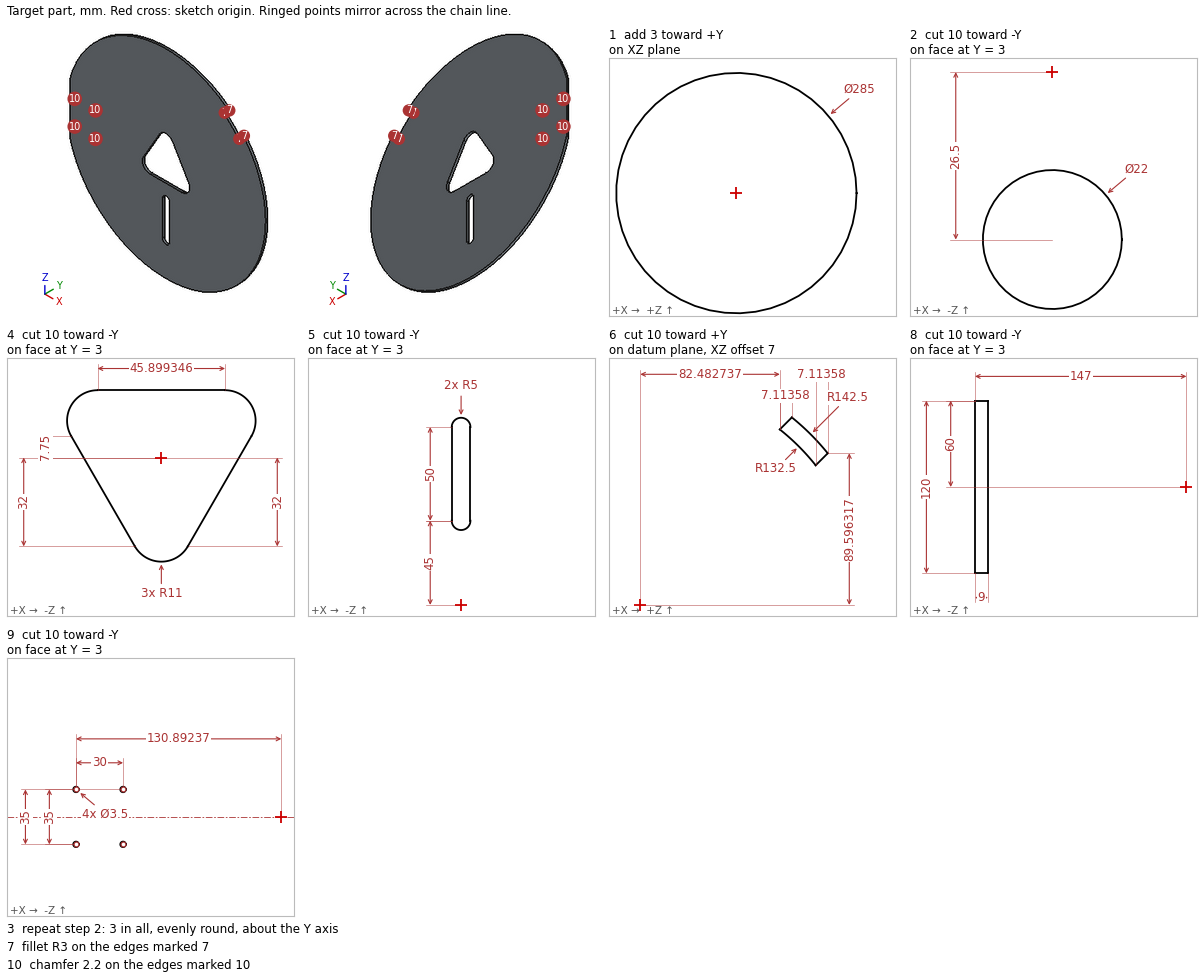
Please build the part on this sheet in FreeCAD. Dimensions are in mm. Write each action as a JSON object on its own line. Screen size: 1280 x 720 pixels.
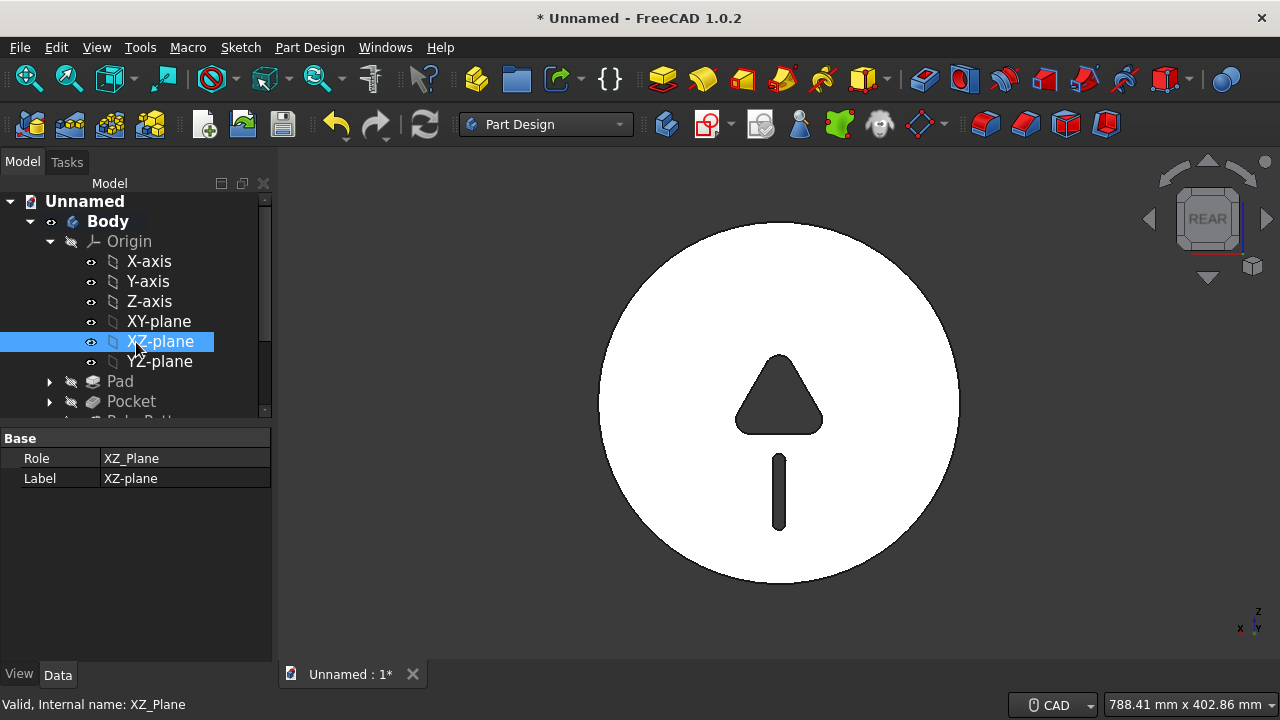
{"action": "left_click", "coordinate": [920, 124]}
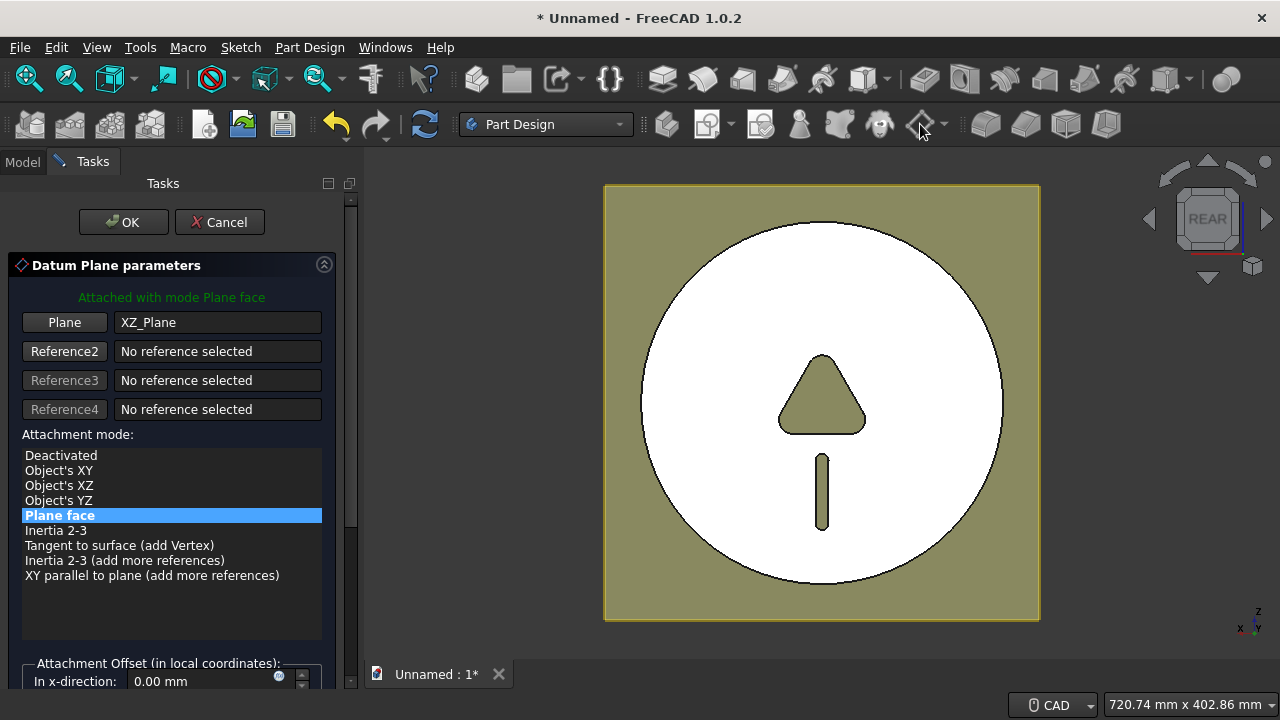
{"action": "scroll", "coordinate": [351, 440], "scroll_direction": "down", "scroll_amount": 3}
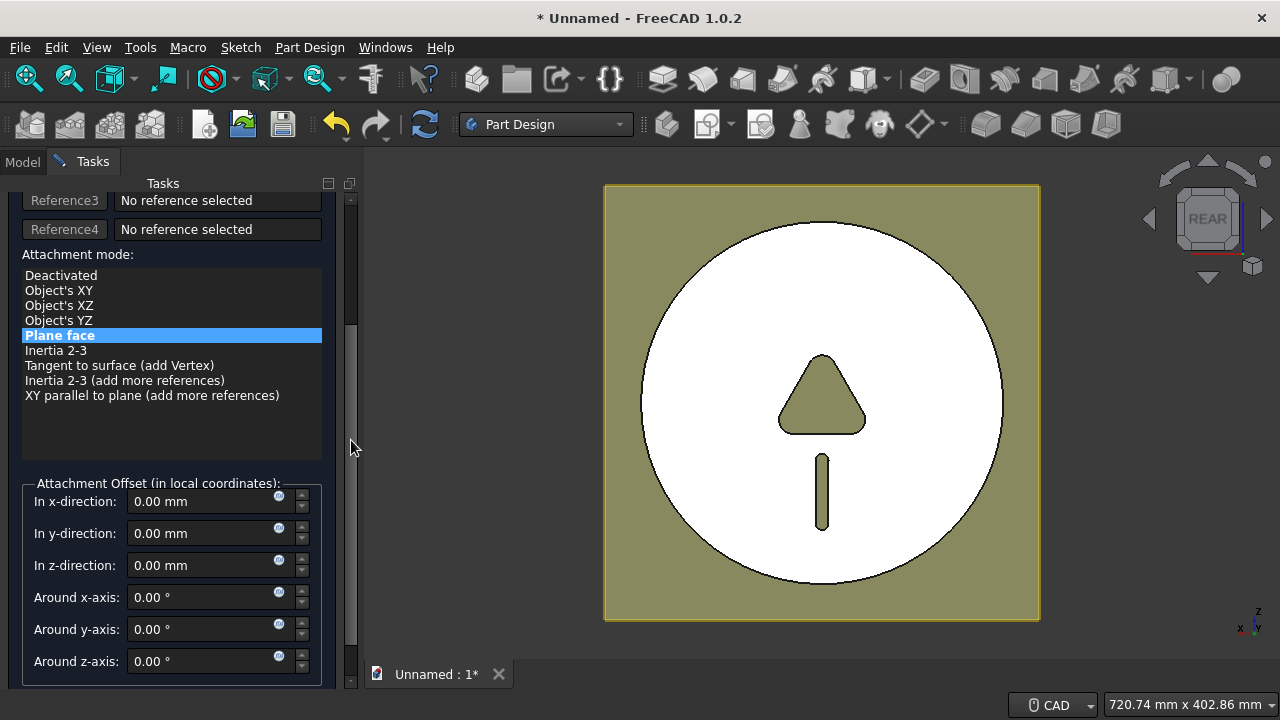
{"action": "triple_click", "coordinate": [210, 565]}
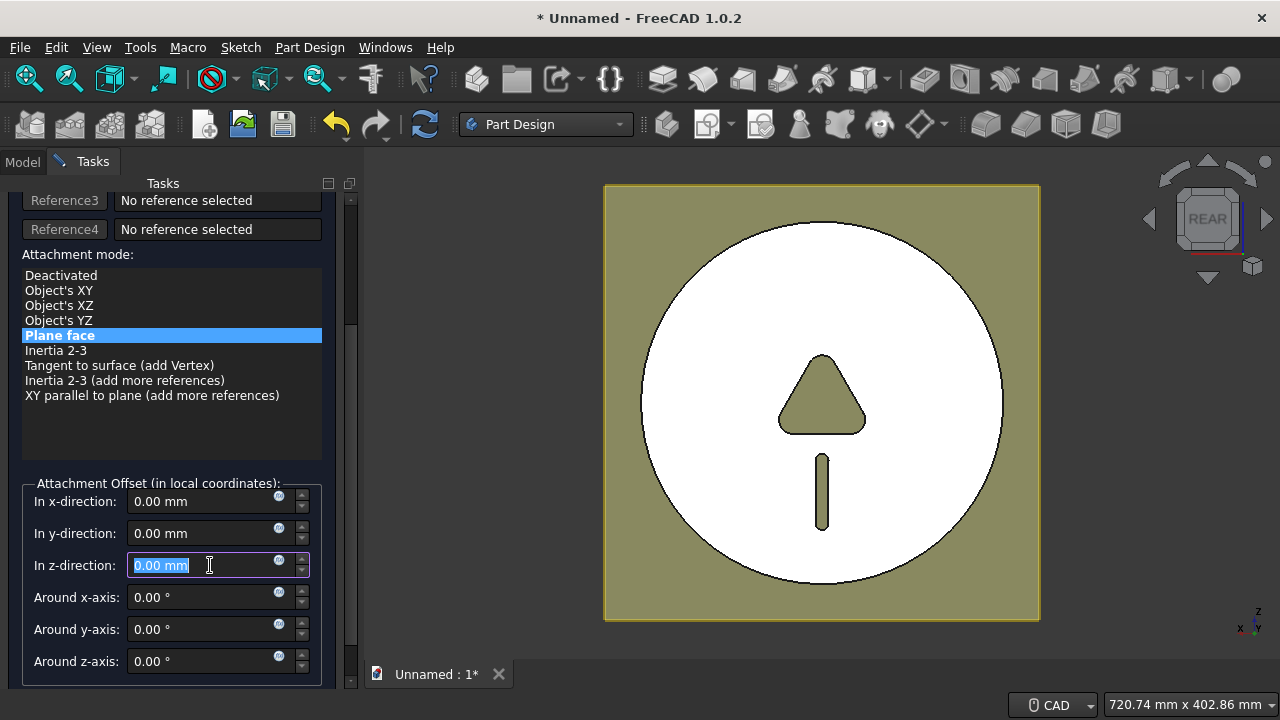
{"action": "type", "text": "7"}
{"action": "key", "text": "Tab"}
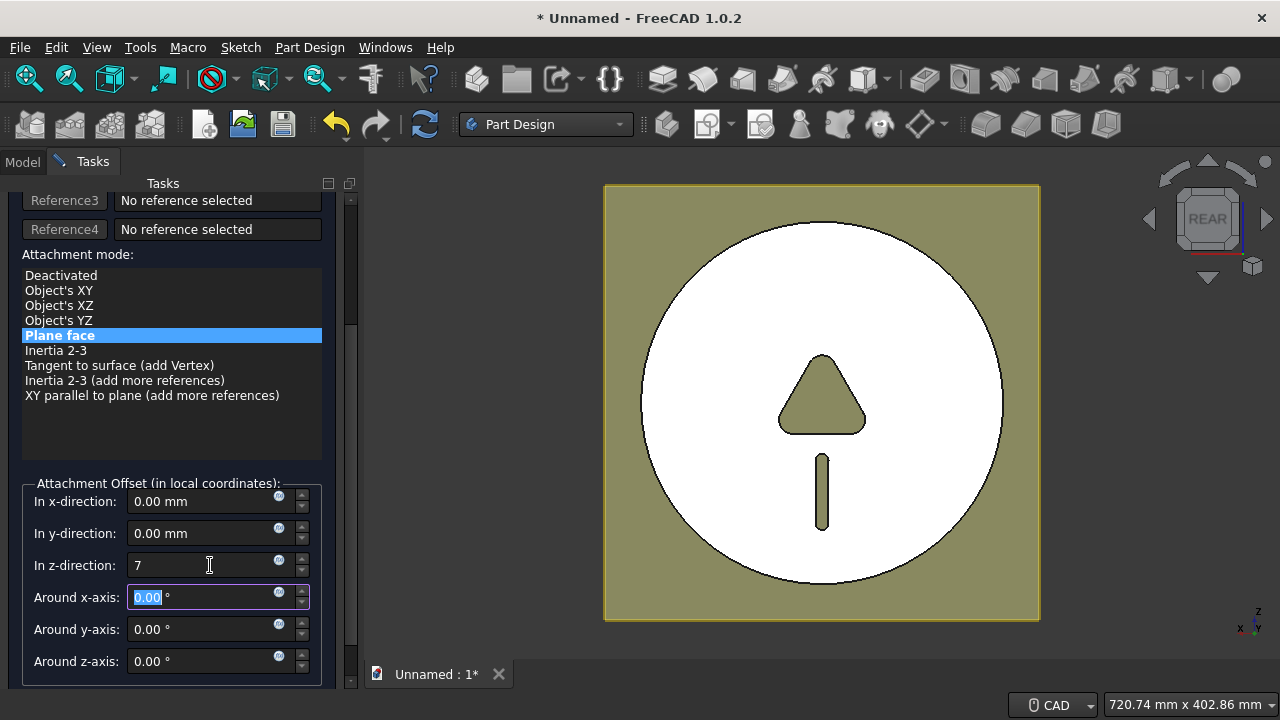
{"action": "scroll", "coordinate": [351, 440], "scroll_direction": "up", "scroll_amount": 4}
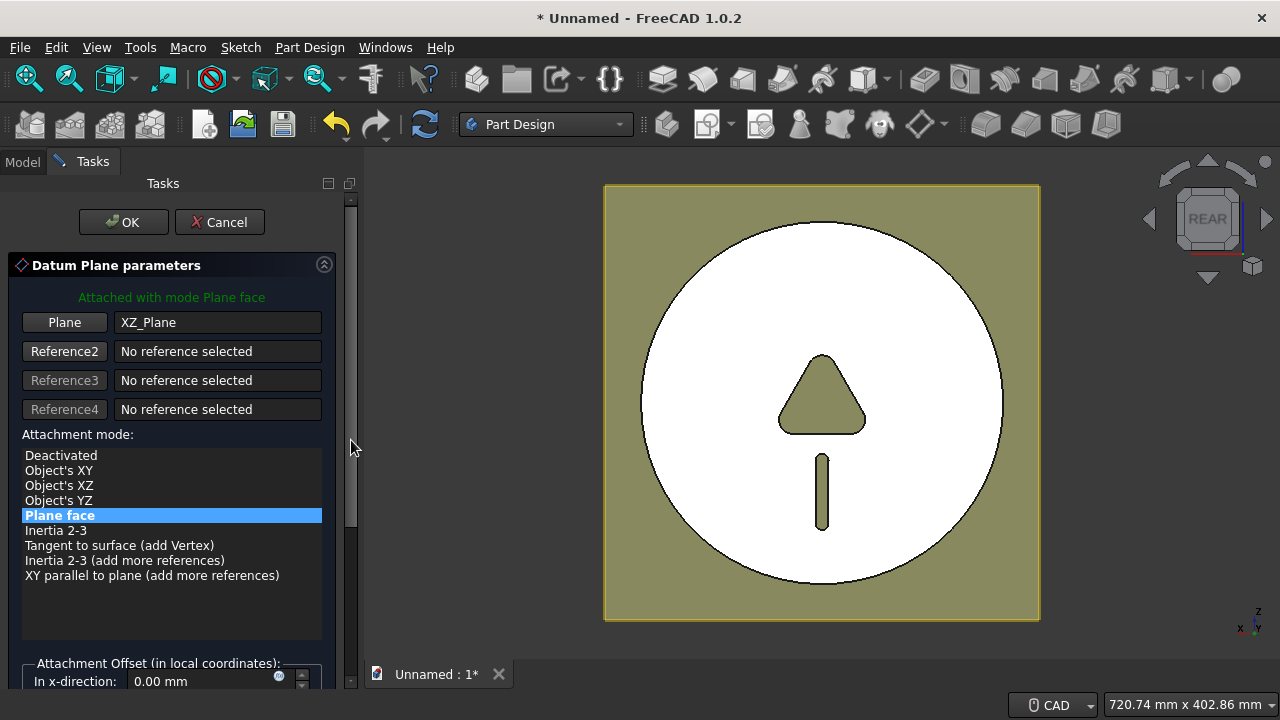
{"action": "left_click", "coordinate": [124, 222]}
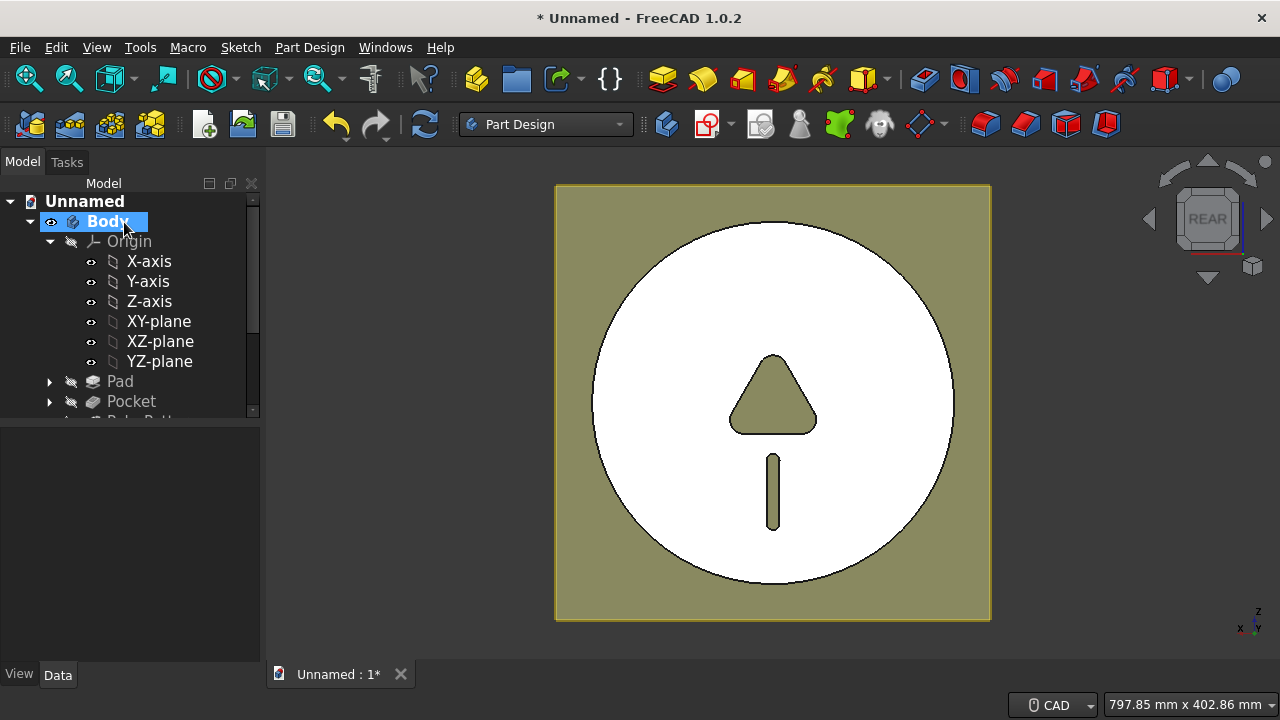
{"action": "scroll", "coordinate": [100, 297], "scroll_direction": "down", "scroll_amount": 3}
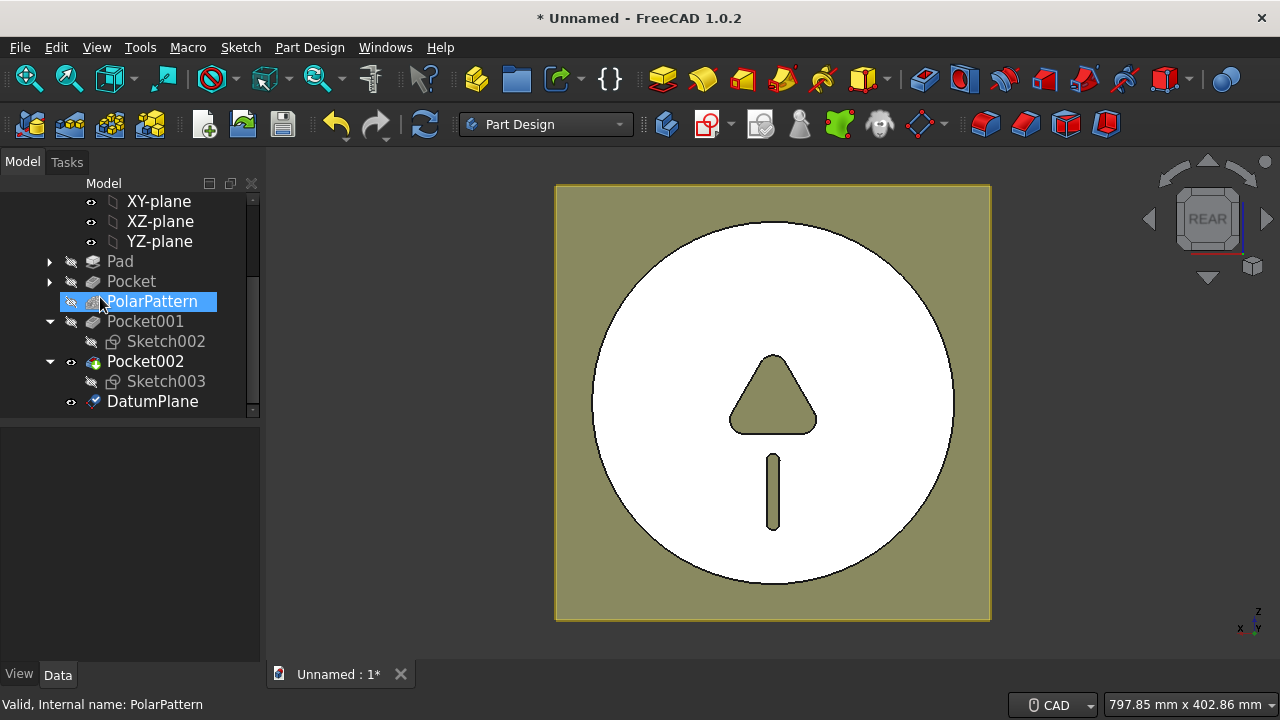
{"action": "left_click", "coordinate": [116, 402]}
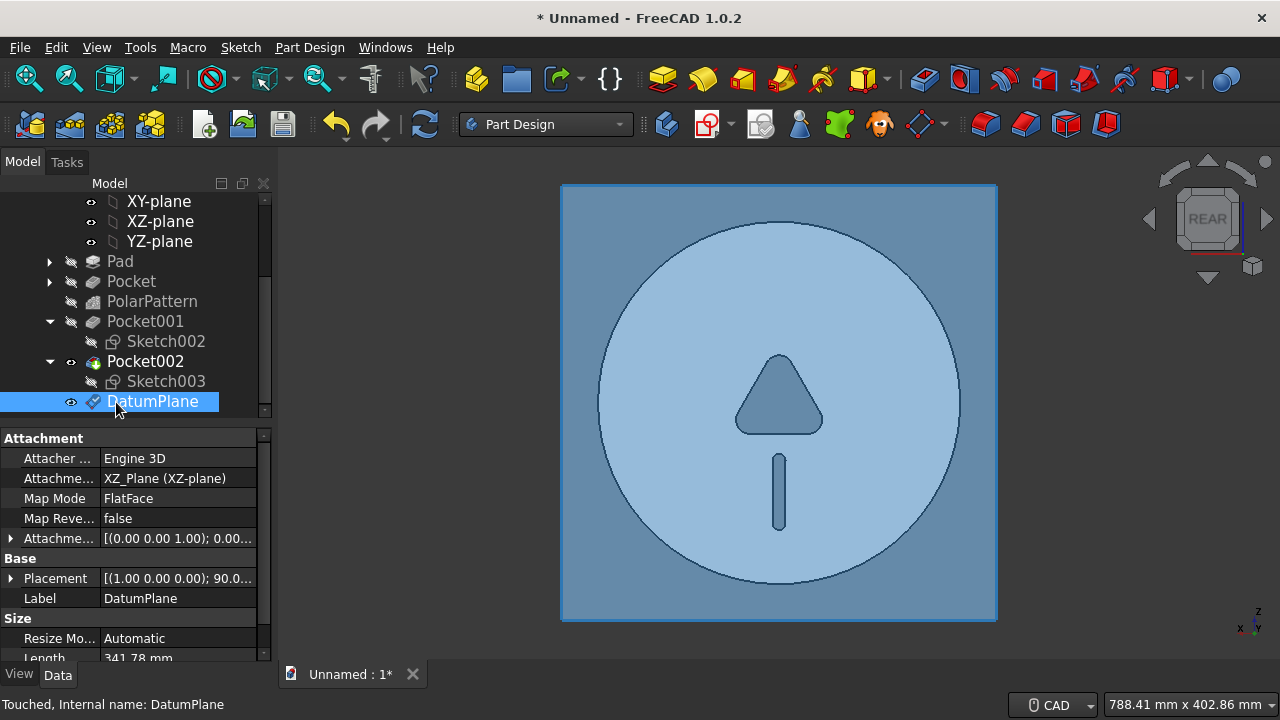
{"action": "left_click", "coordinate": [708, 124]}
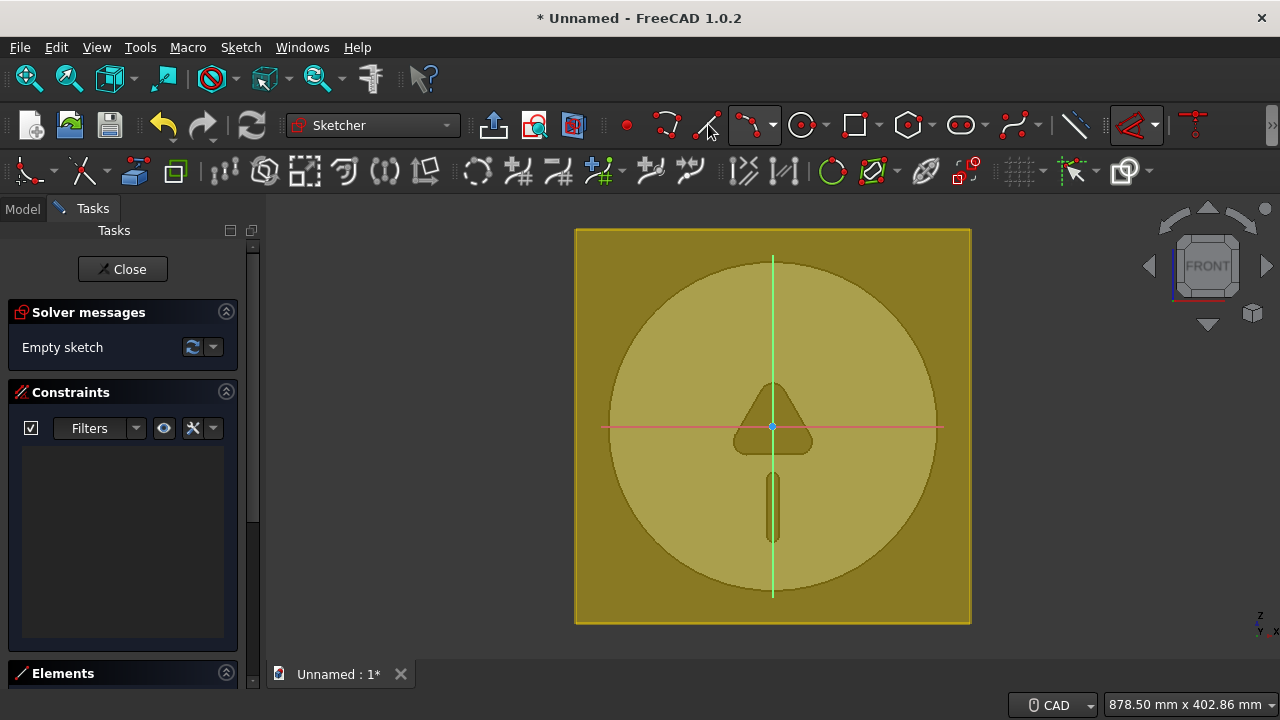
{"action": "scroll", "coordinate": [907, 301], "scroll_direction": "up", "scroll_amount": 11}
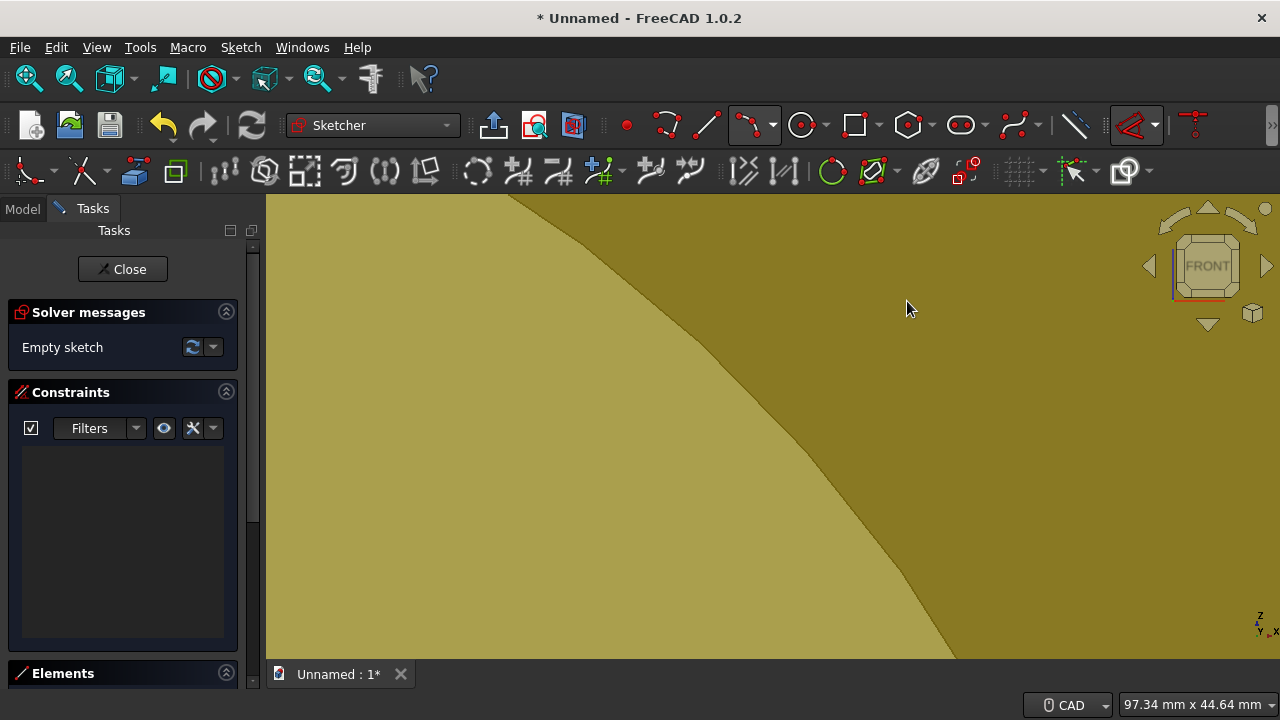
{"action": "left_click", "coordinate": [708, 126]}